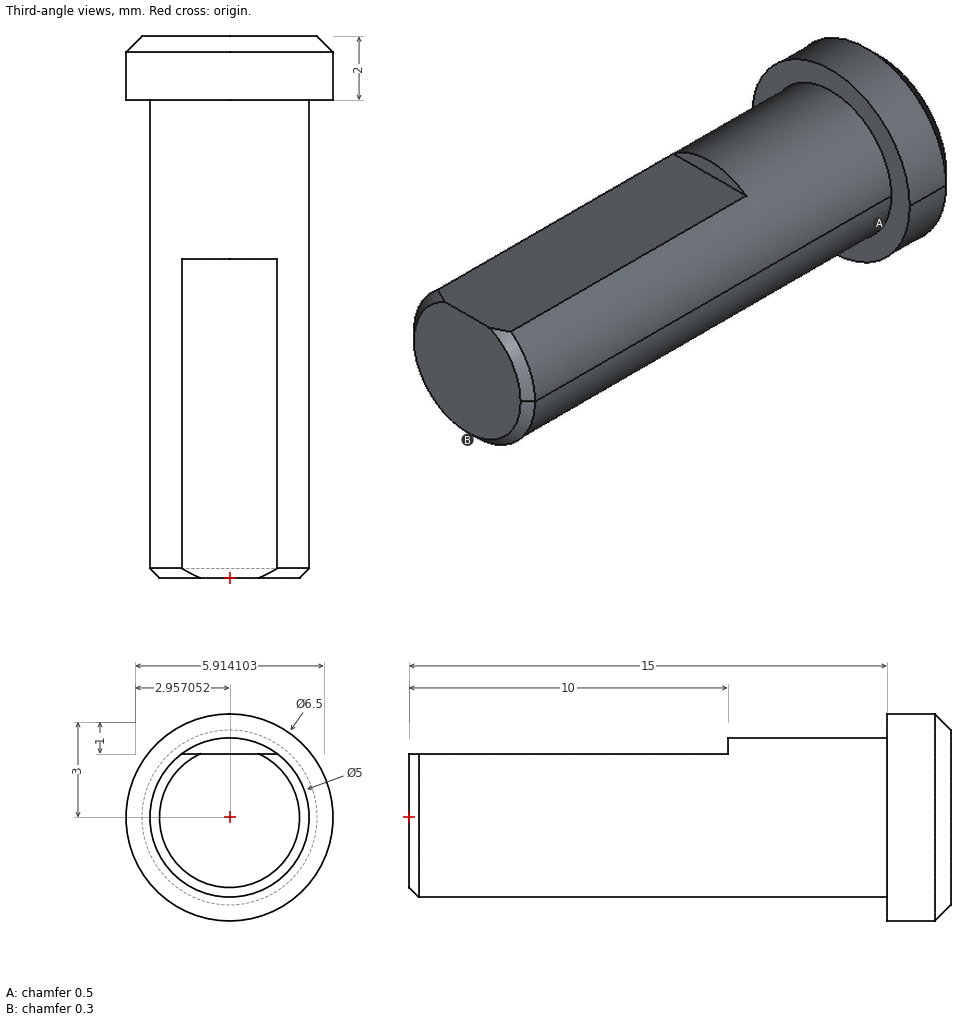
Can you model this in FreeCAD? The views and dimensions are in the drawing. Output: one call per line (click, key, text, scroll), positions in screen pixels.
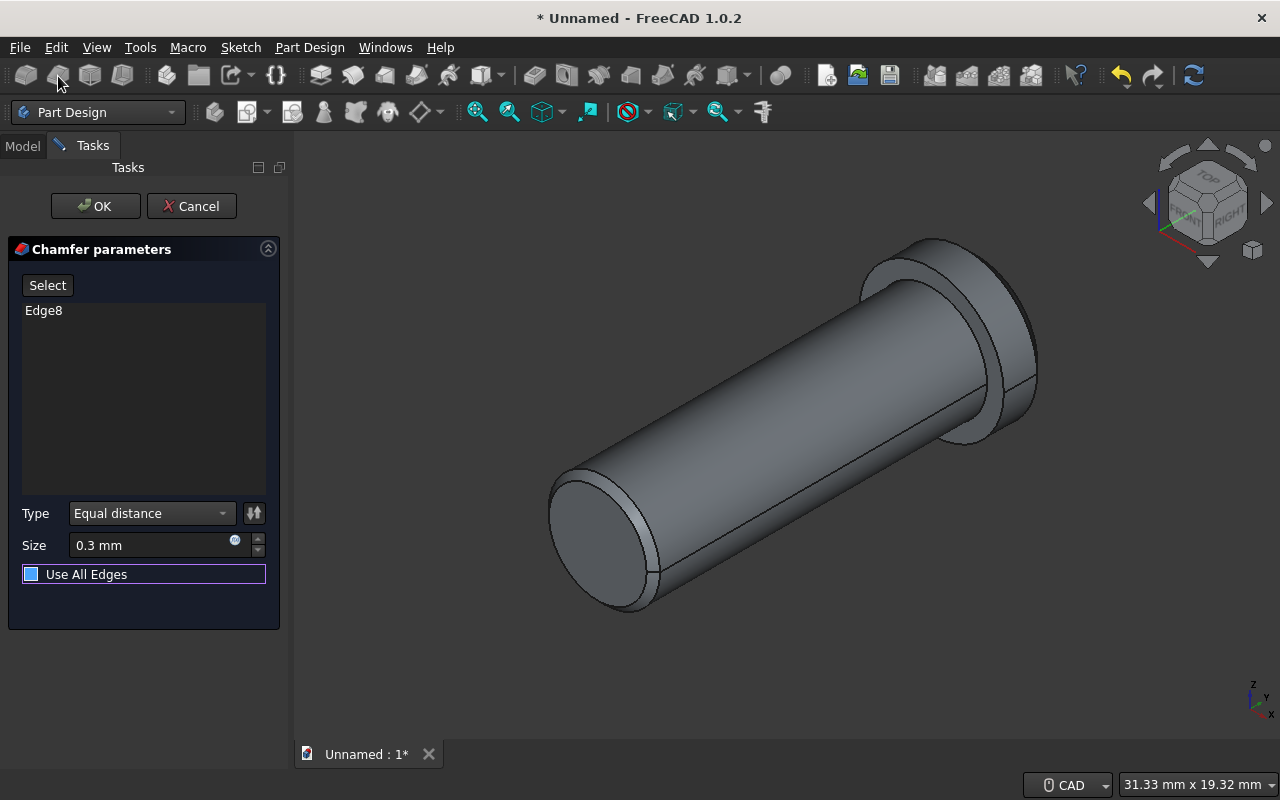
click(96, 206)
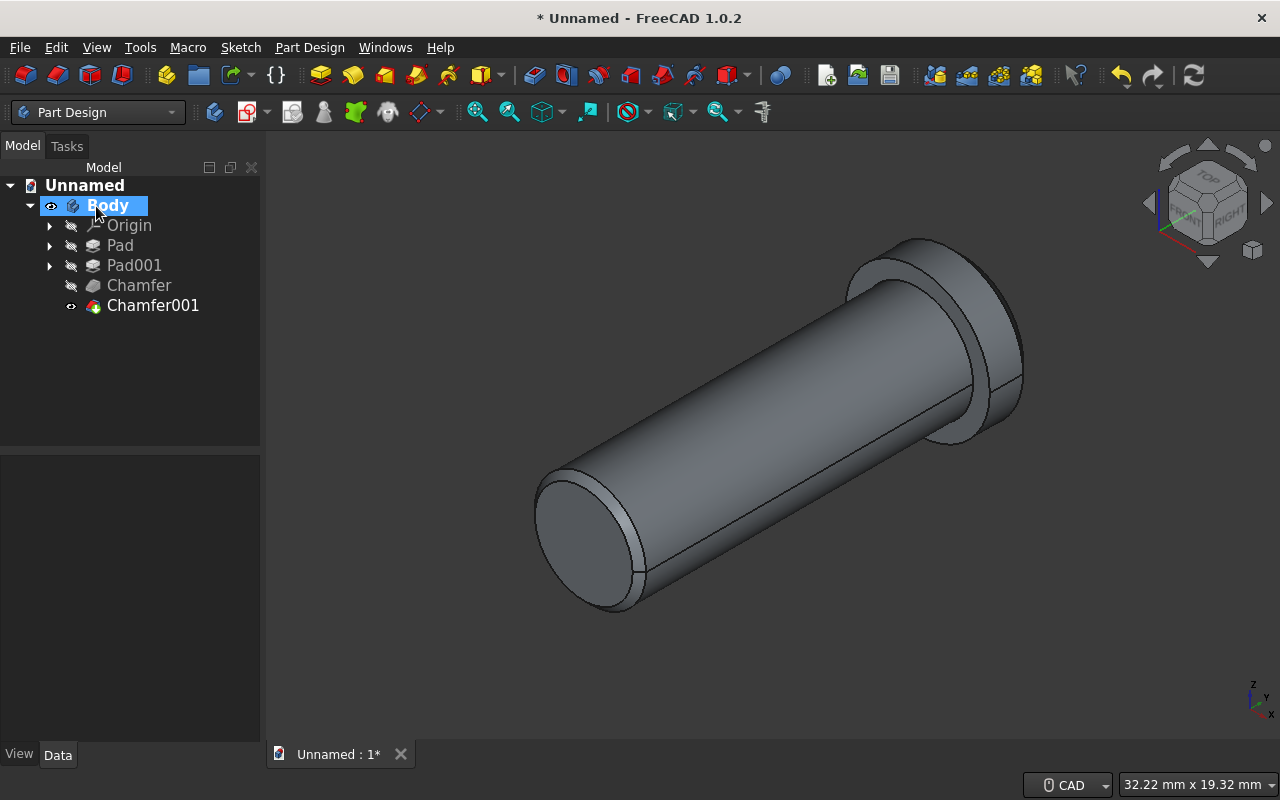
click(584, 543)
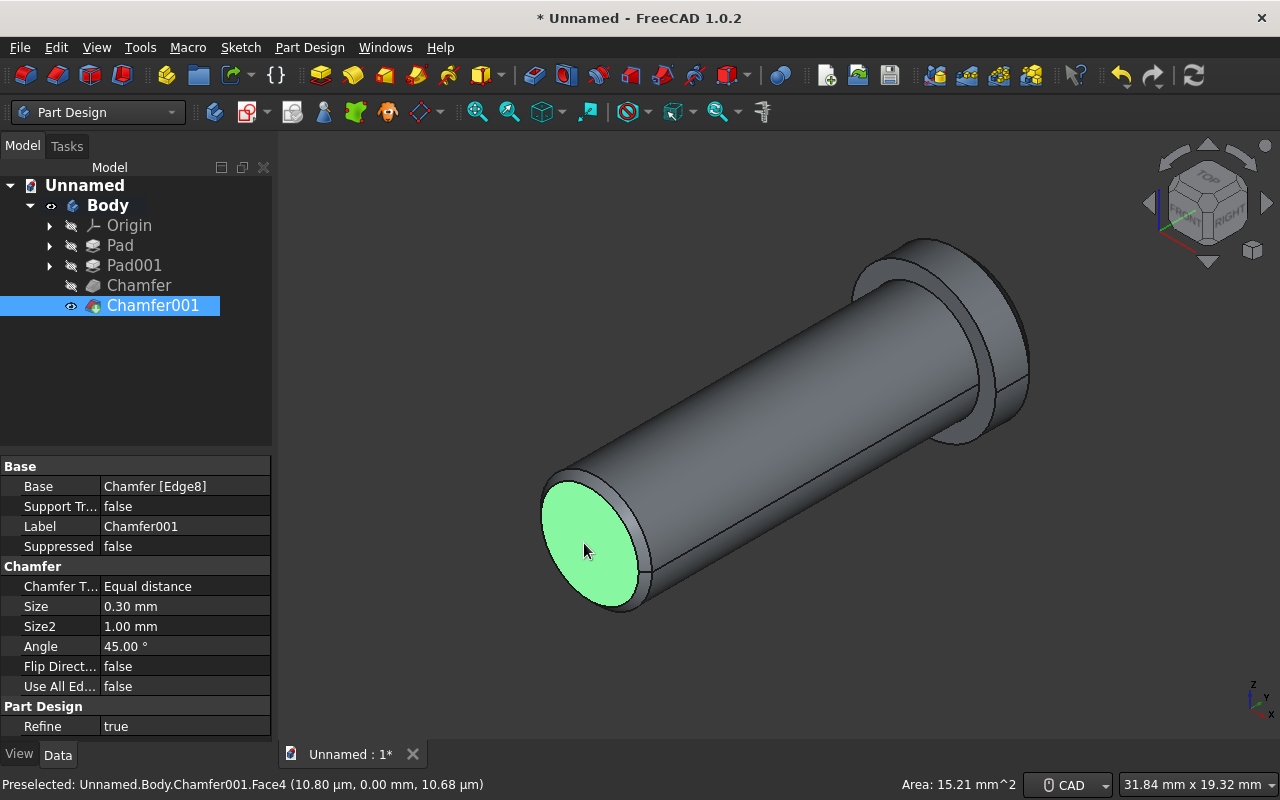
click(248, 112)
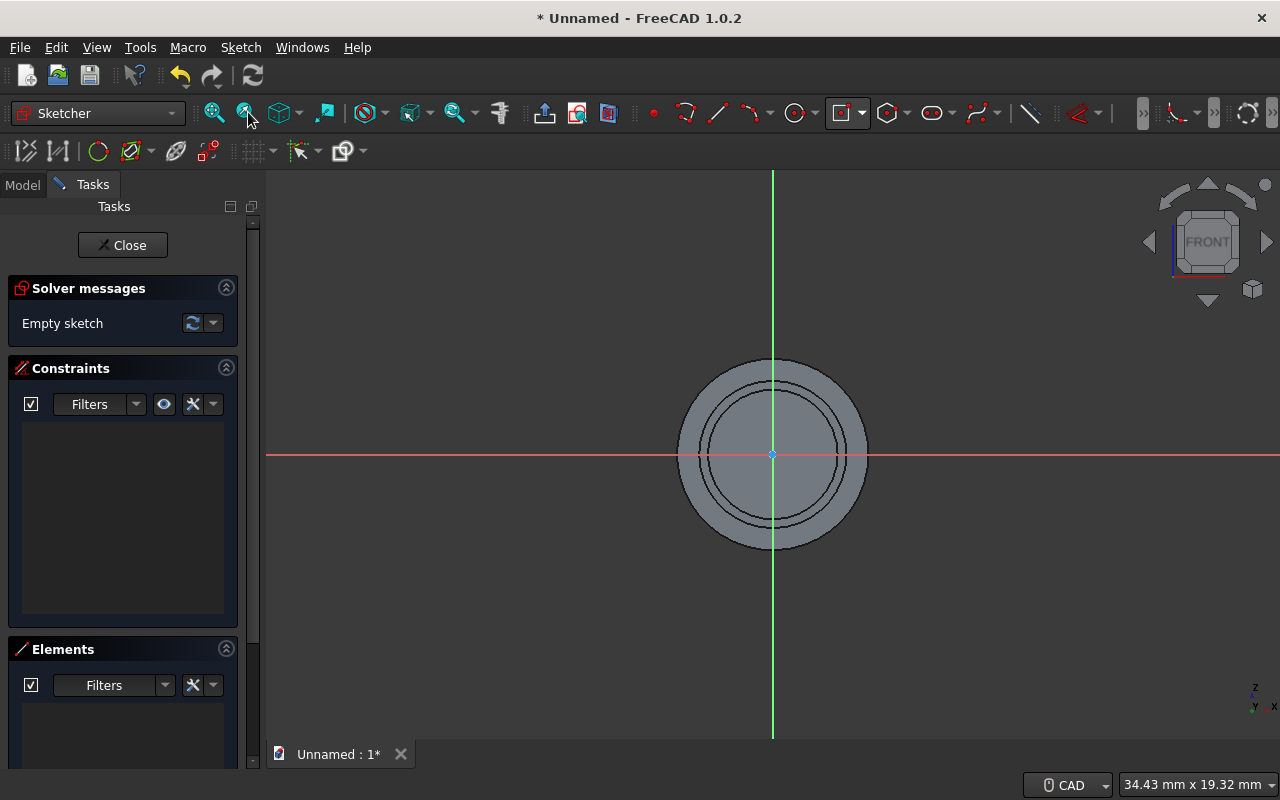
scroll(802, 391, up, 6)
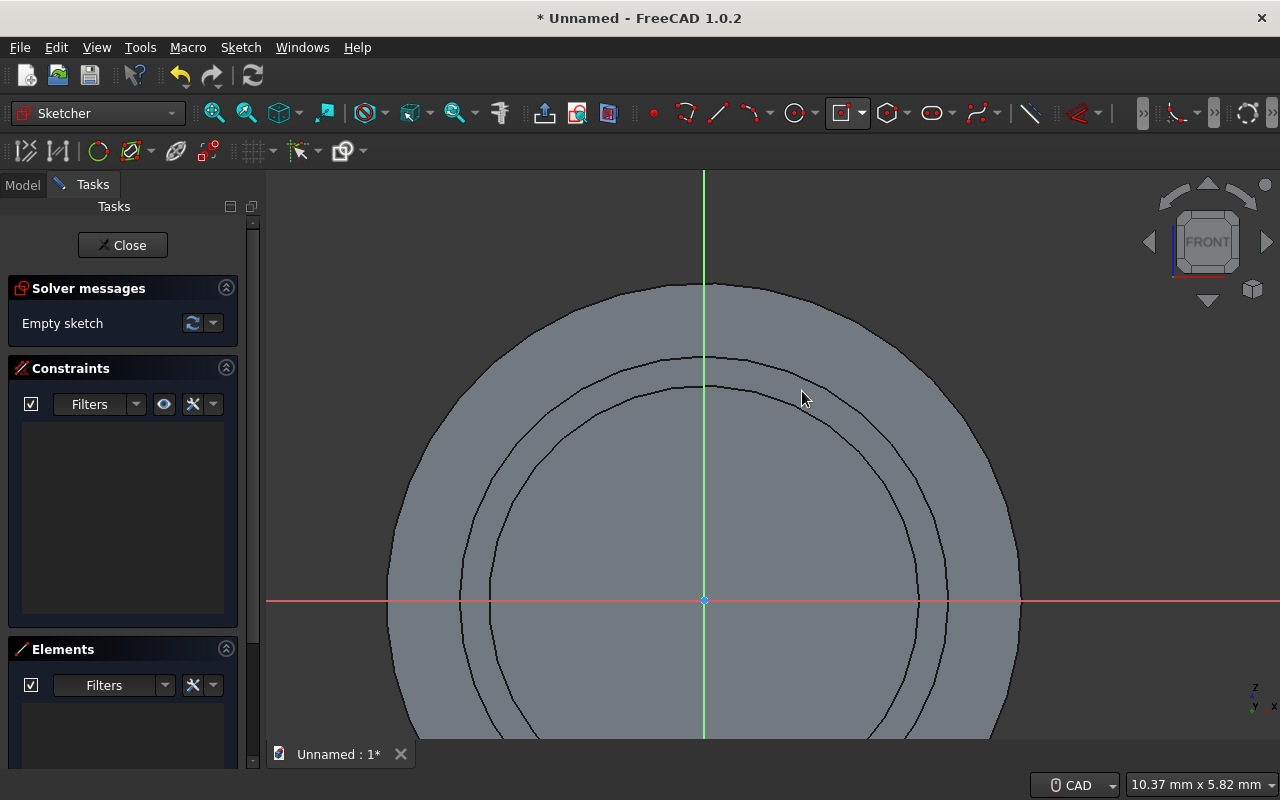
key(g)
key(r)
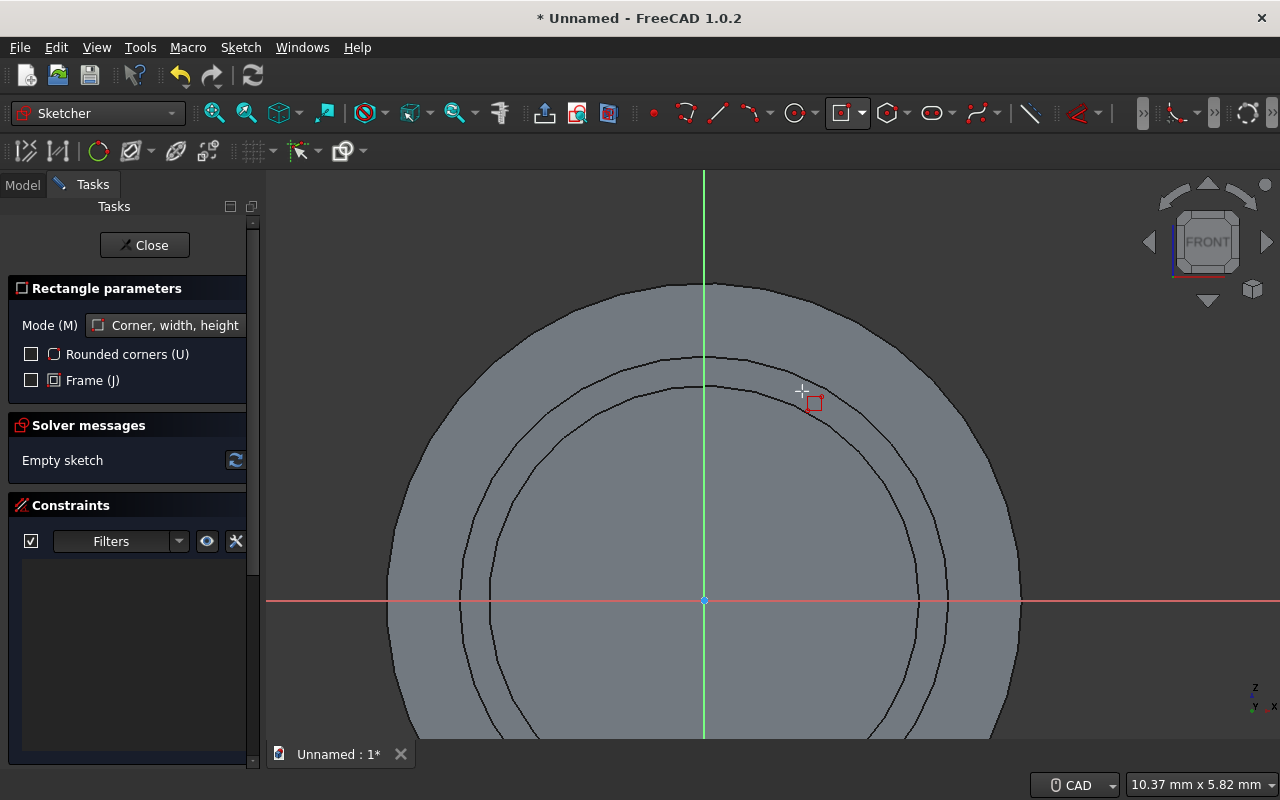
click(415, 308)
click(993, 405)
key(Escape)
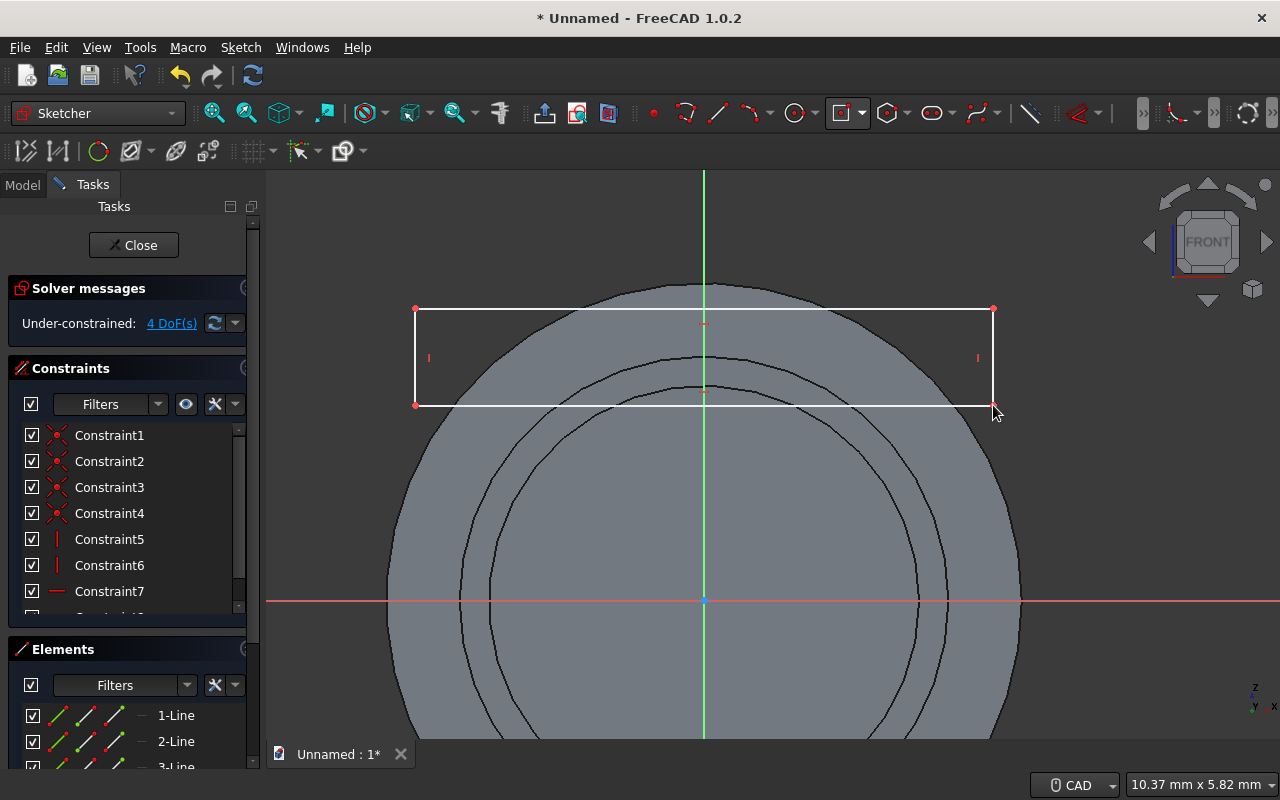
click(1078, 114)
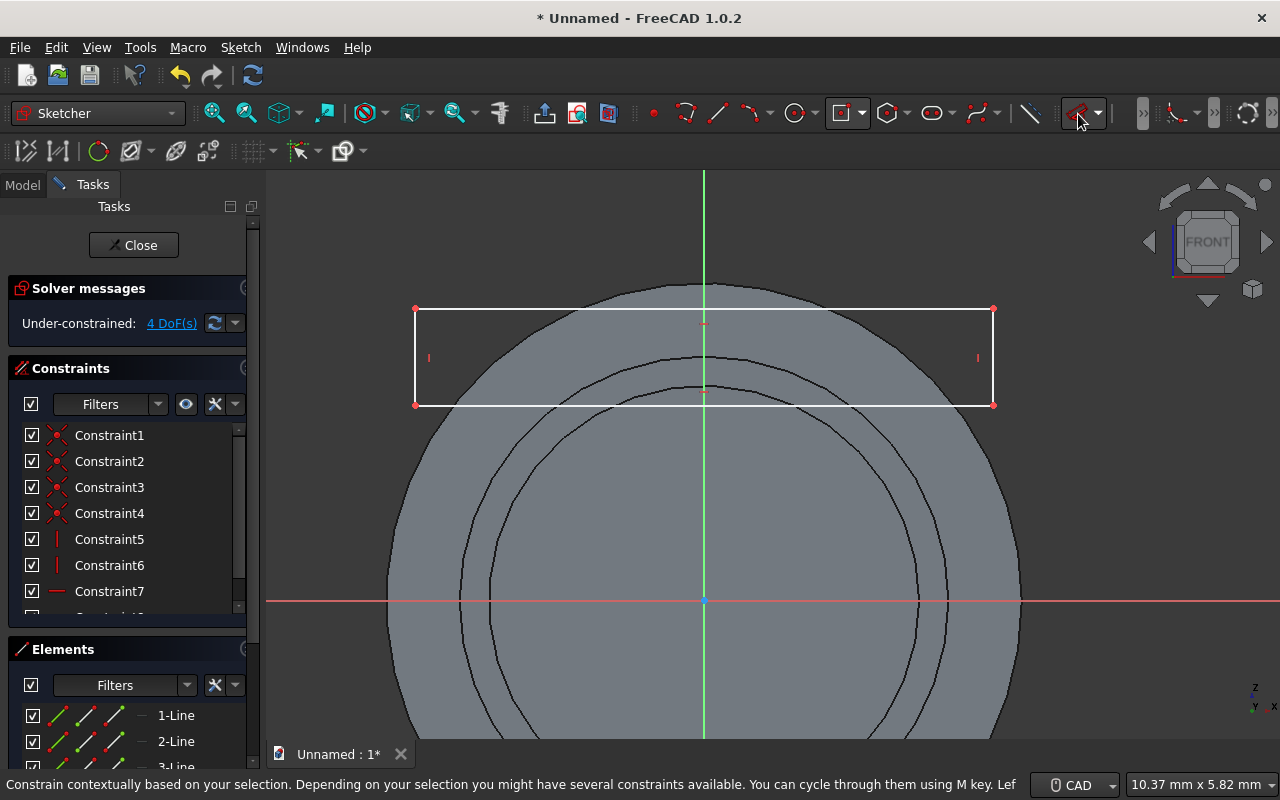
click(415, 338)
click(381, 357)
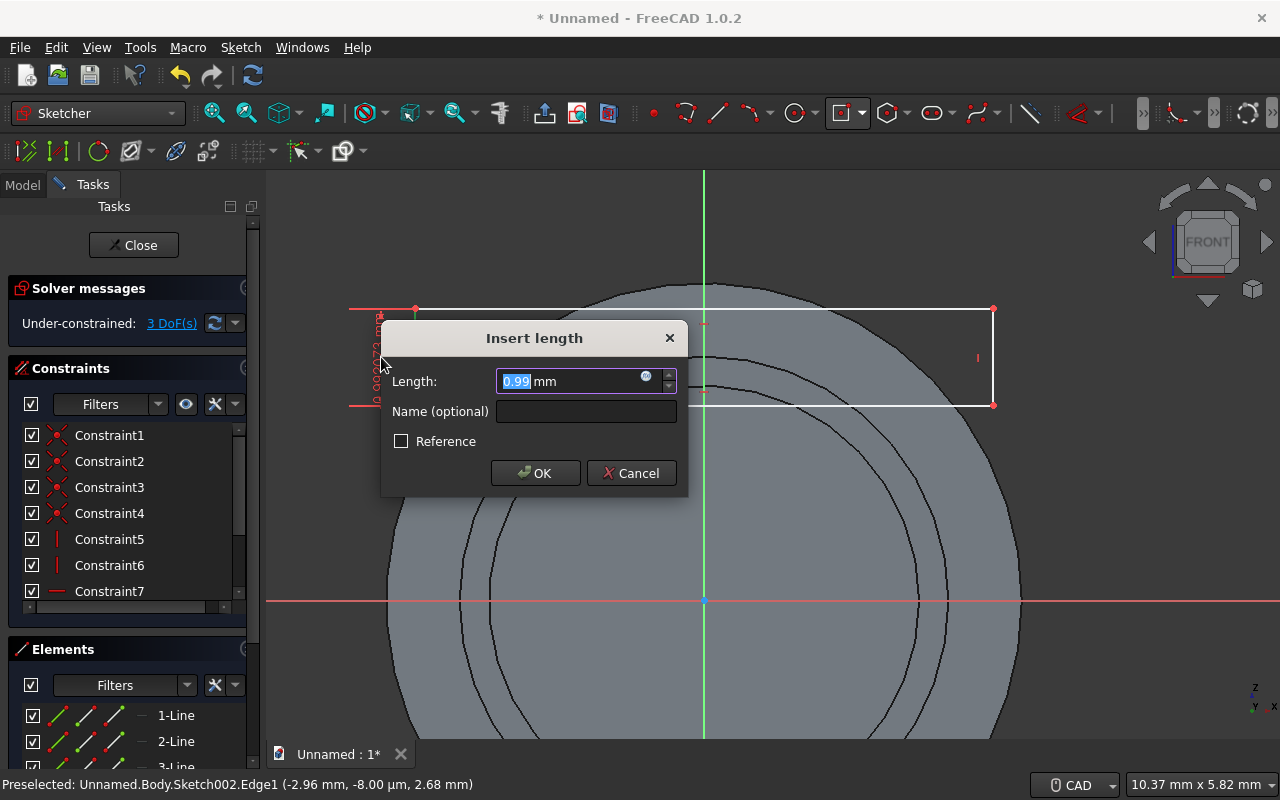
text(1)
key(Return)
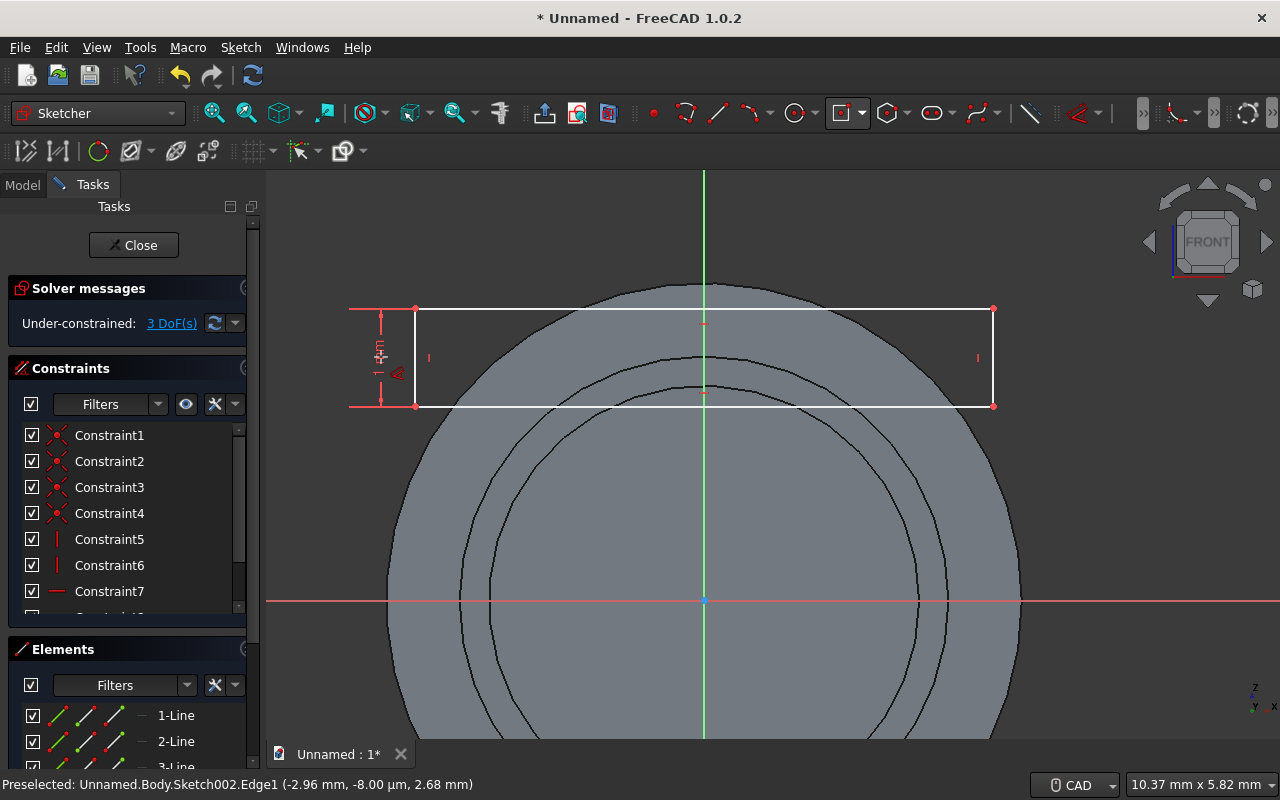
click(415, 309)
click(381, 455)